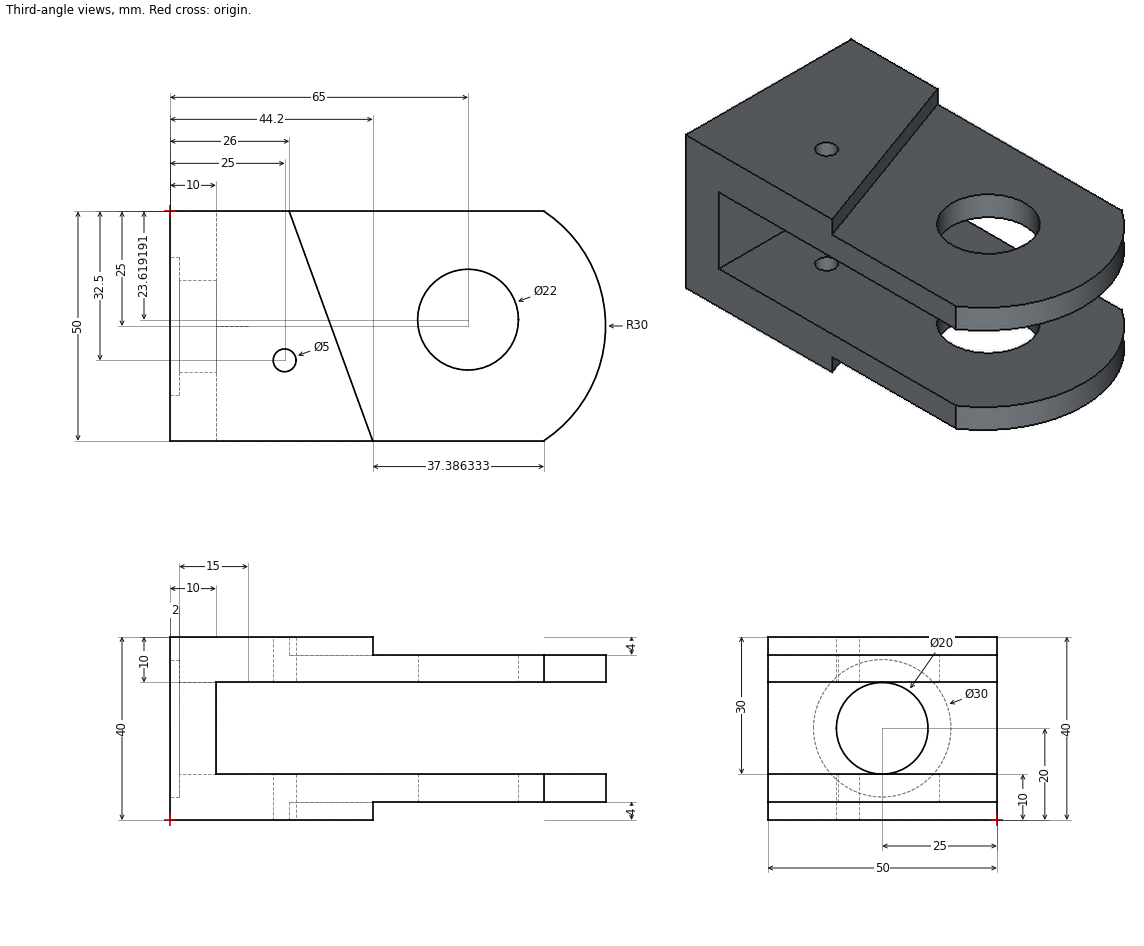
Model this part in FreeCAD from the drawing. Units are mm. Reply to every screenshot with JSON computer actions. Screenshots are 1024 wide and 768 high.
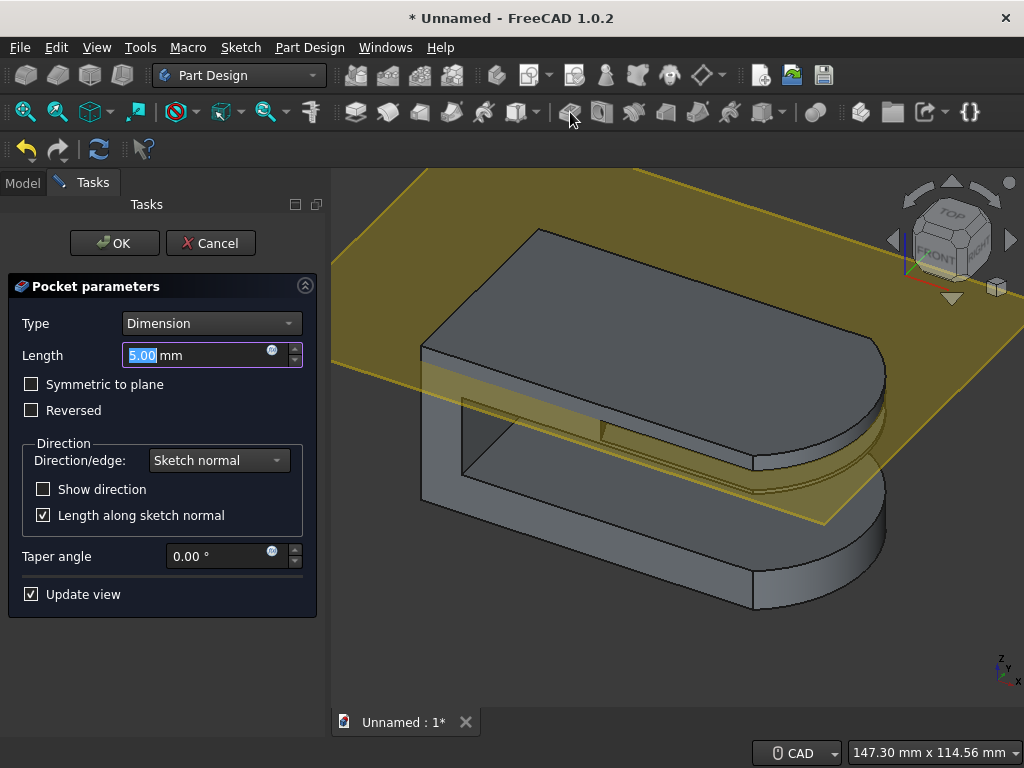
{"action": "type", "text": "4"}
{"action": "key", "text": "Tab"}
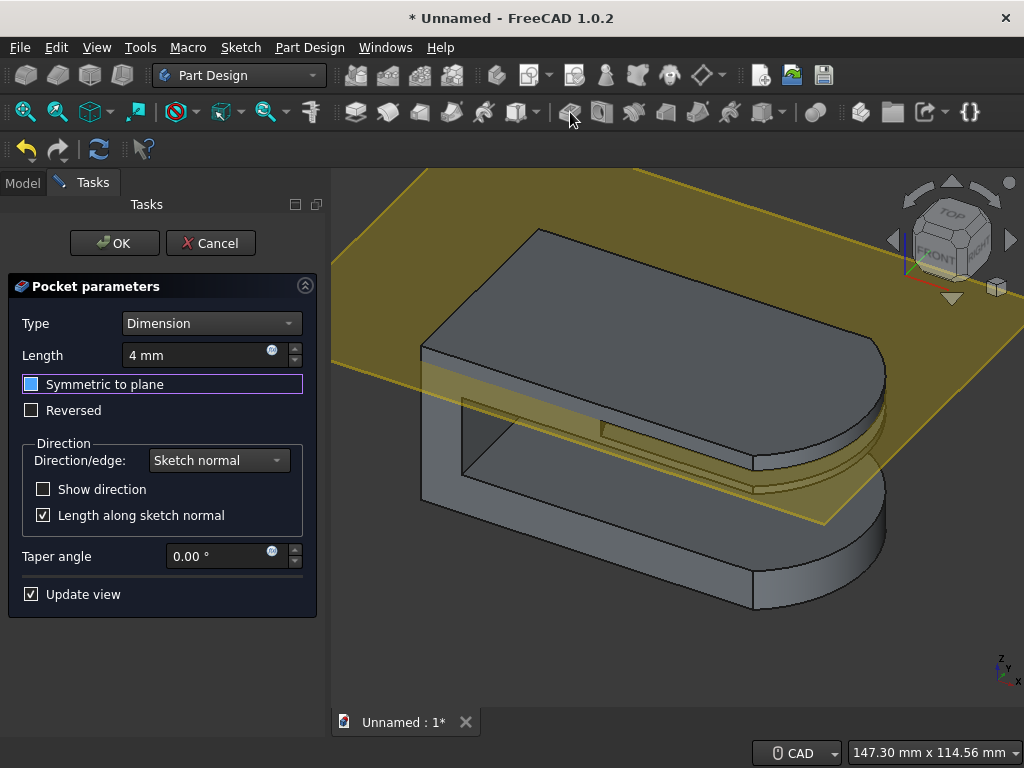
{"action": "left_click", "coordinate": [30, 410]}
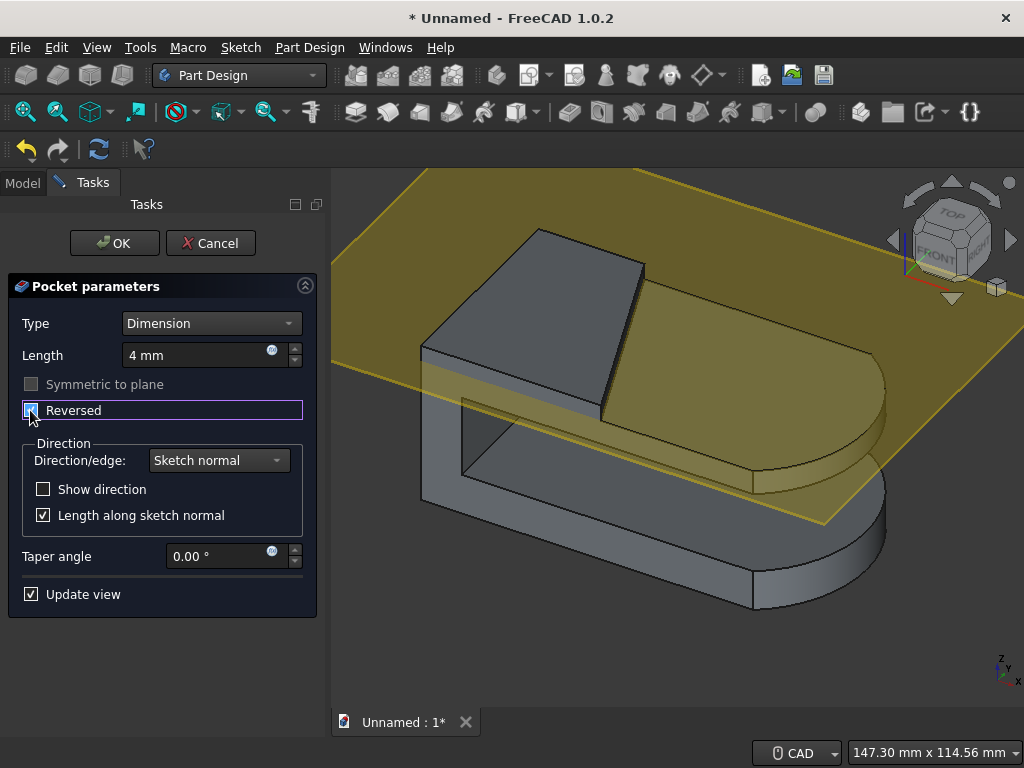
{"action": "left_click", "coordinate": [115, 243]}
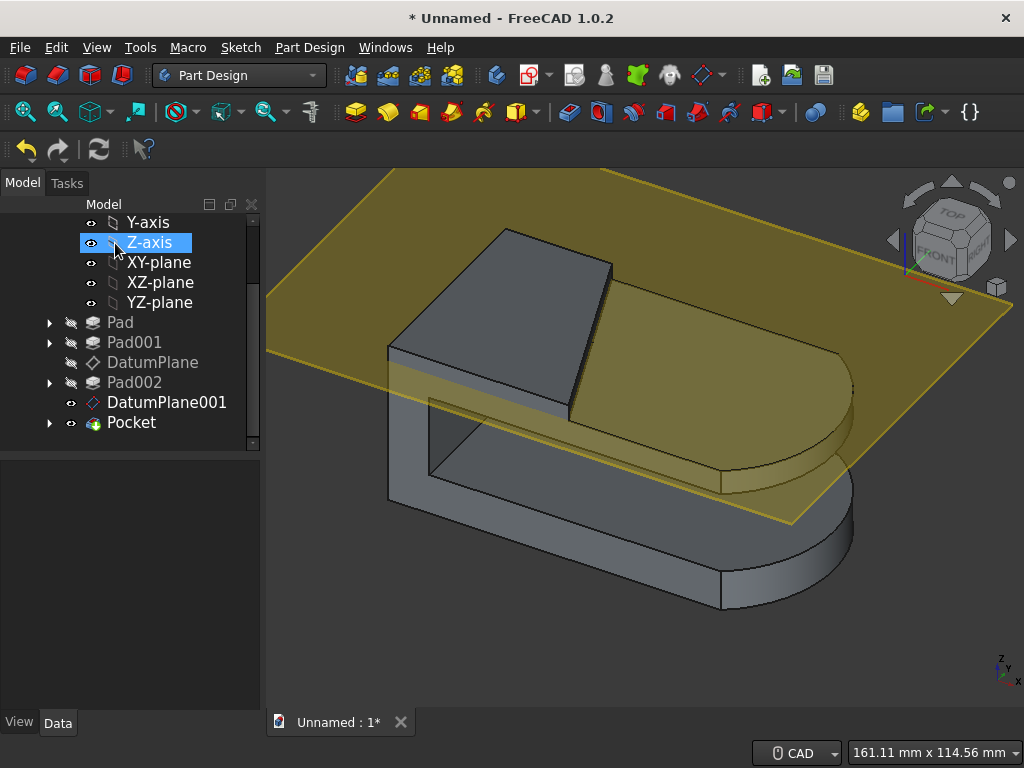
{"action": "left_click", "coordinate": [116, 403]}
{"action": "key", "text": "space"}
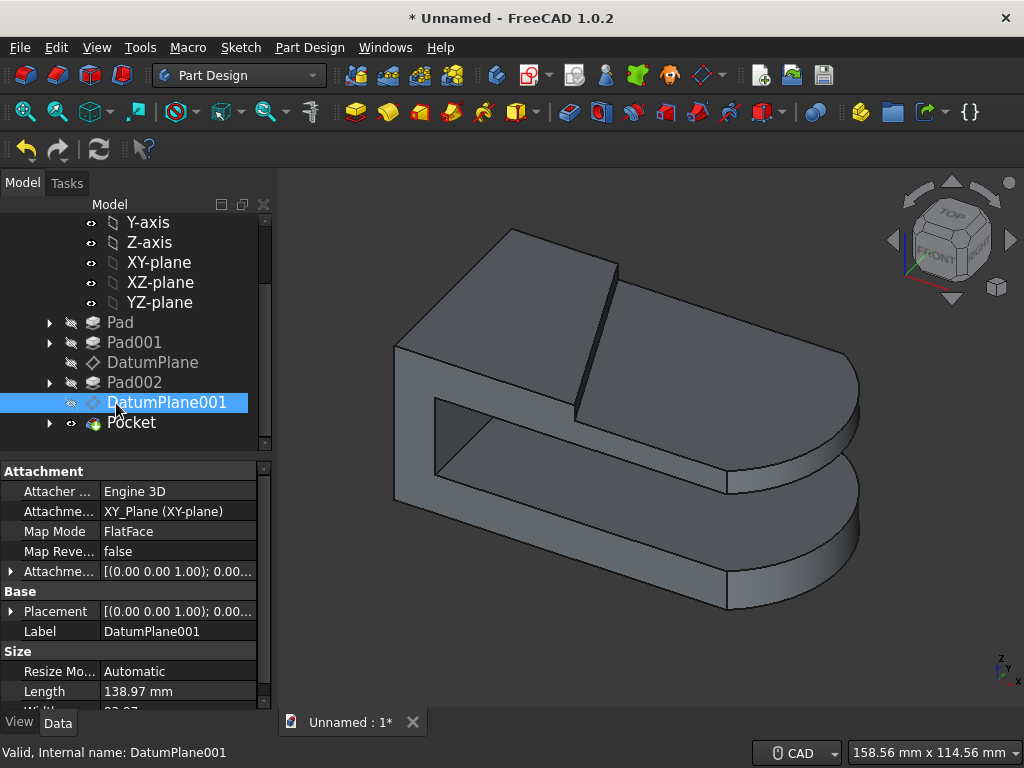
{"action": "left_click", "coordinate": [318, 667]}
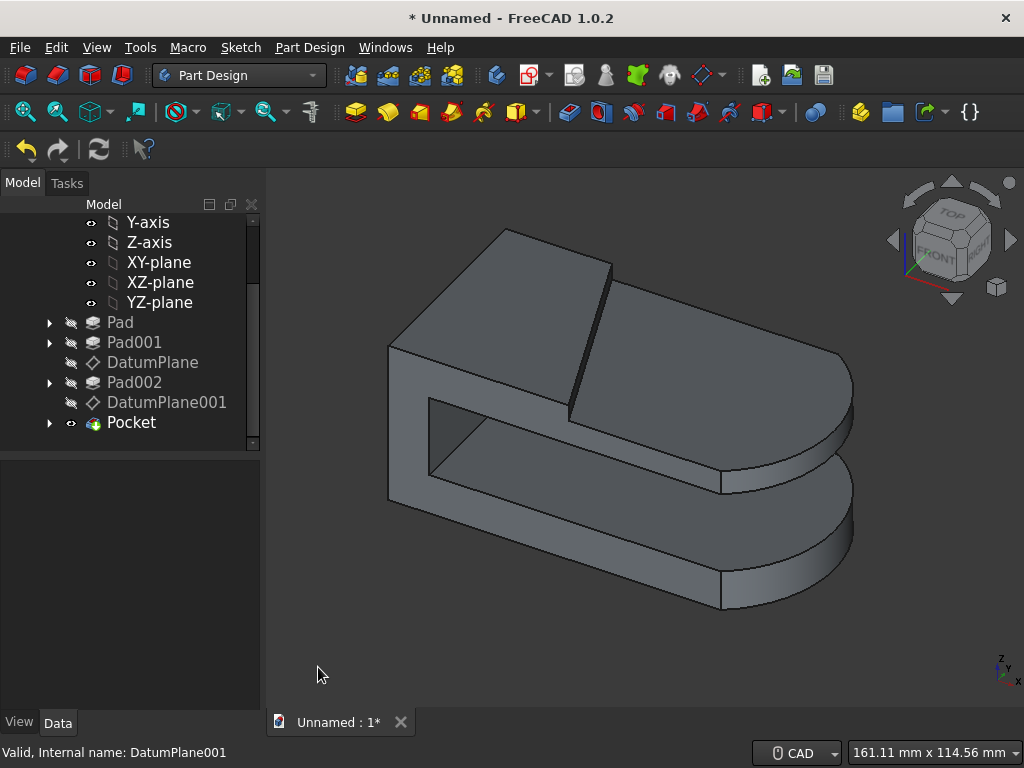
{"action": "left_click", "coordinate": [530, 76]}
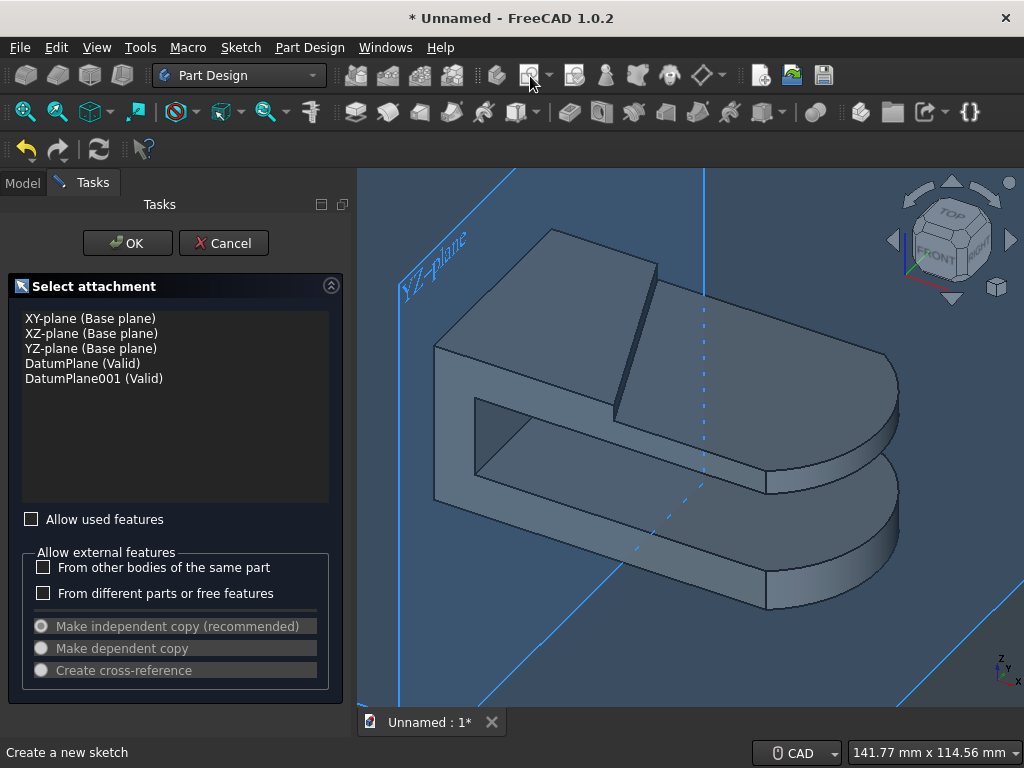
{"action": "left_click", "coordinate": [82, 318]}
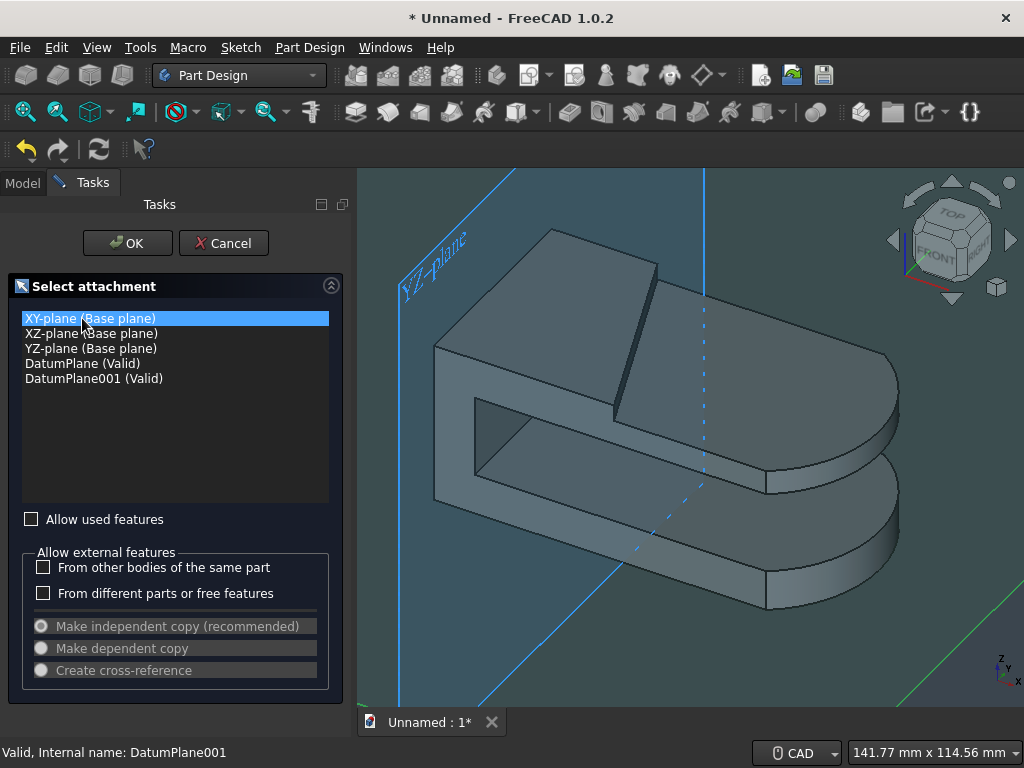
{"action": "left_click", "coordinate": [128, 243]}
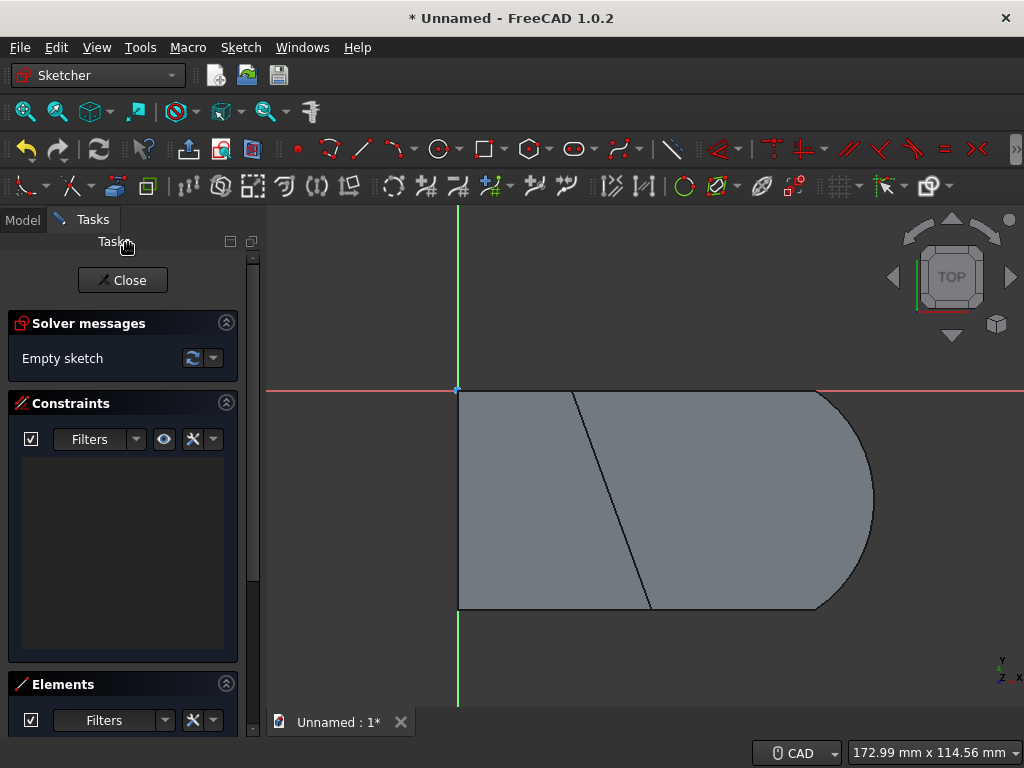
{"action": "left_click", "coordinate": [254, 150]}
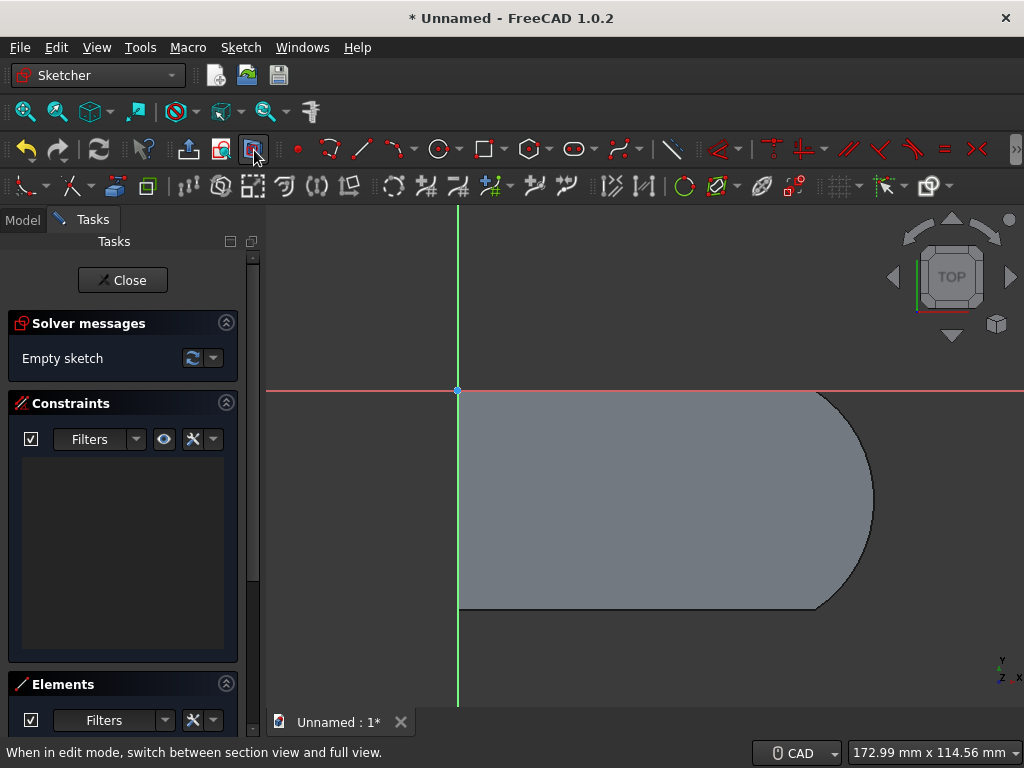
{"action": "scroll", "coordinate": [294, 256], "scroll_direction": "down", "scroll_amount": 1}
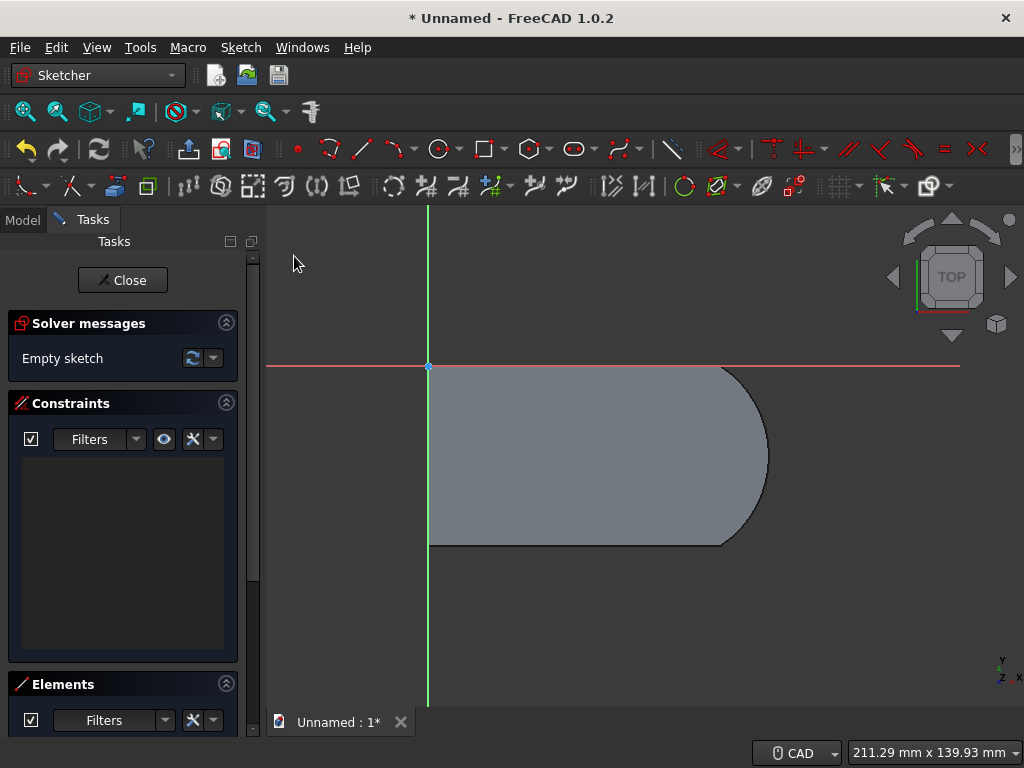
{"action": "key", "text": "g m"}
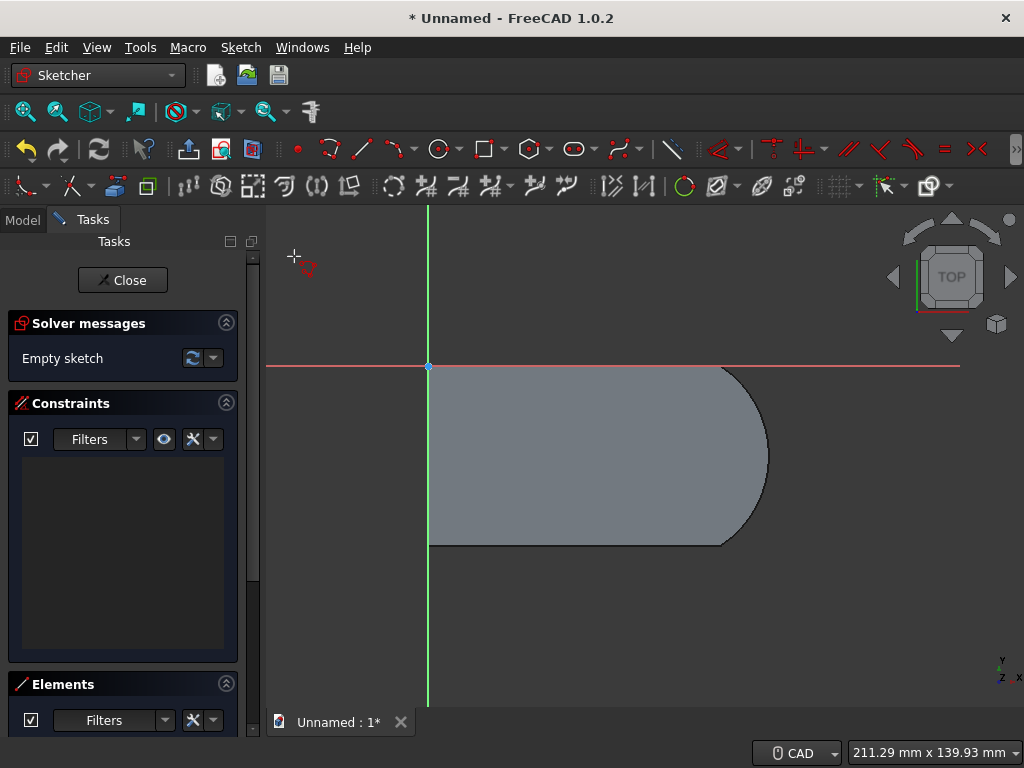
{"action": "left_click", "coordinate": [721, 546]}
{"action": "left_click", "coordinate": [587, 546]}
{"action": "left_click", "coordinate": [521, 366]}
{"action": "left_click", "coordinate": [721, 375]}
{"action": "right_click", "coordinate": [721, 375]}